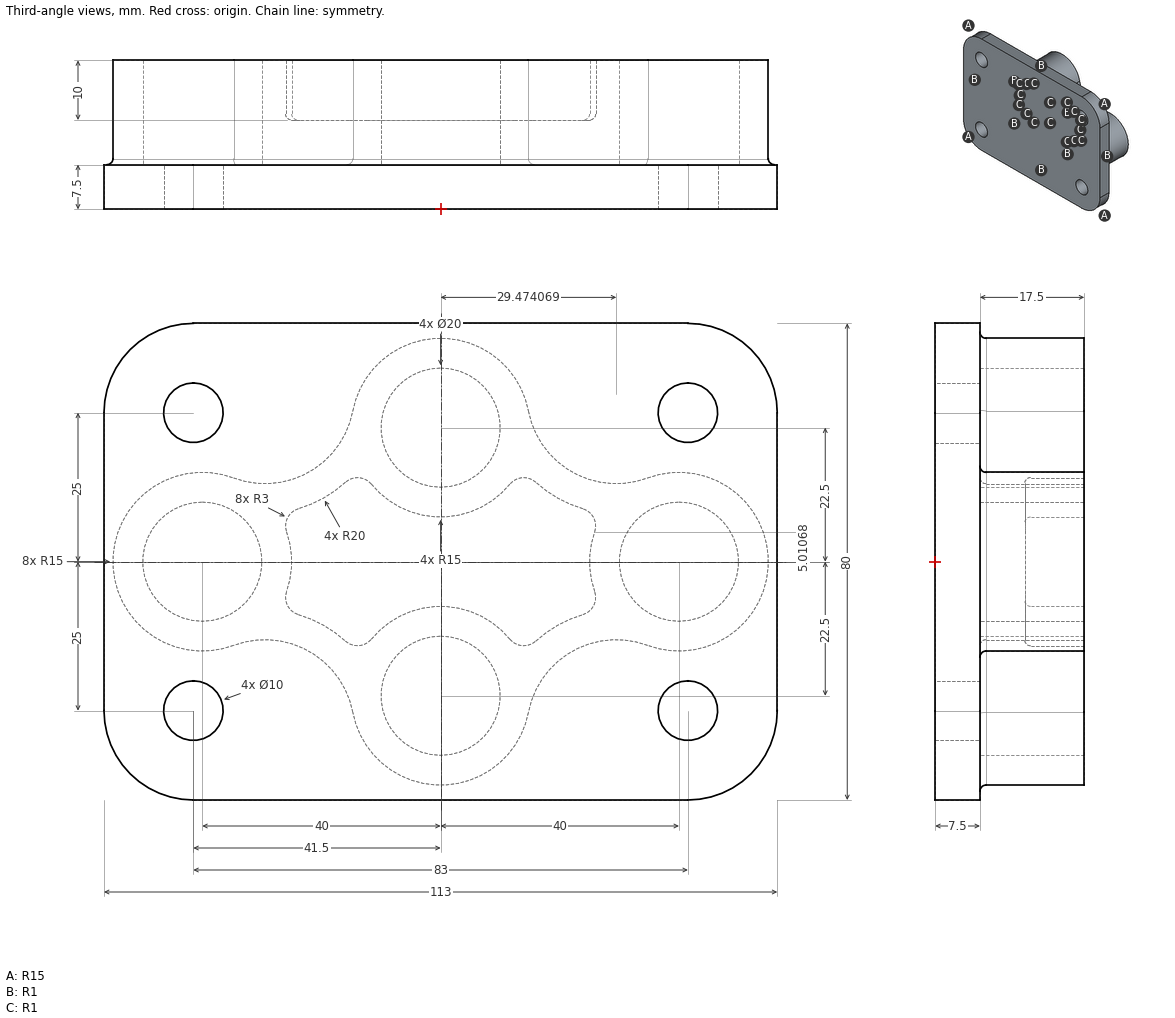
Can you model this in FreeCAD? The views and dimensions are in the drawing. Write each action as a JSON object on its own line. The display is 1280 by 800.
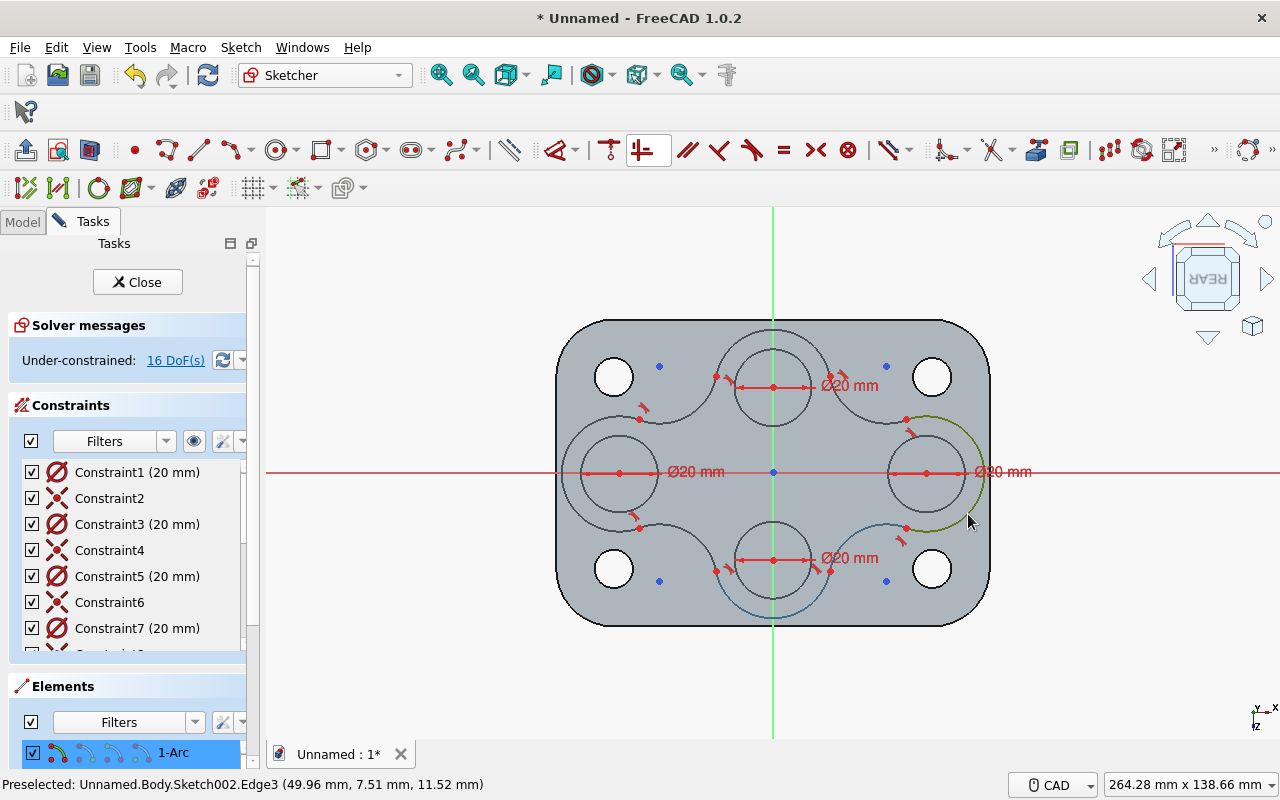
{"action": "left_click", "coordinate": [843, 404]}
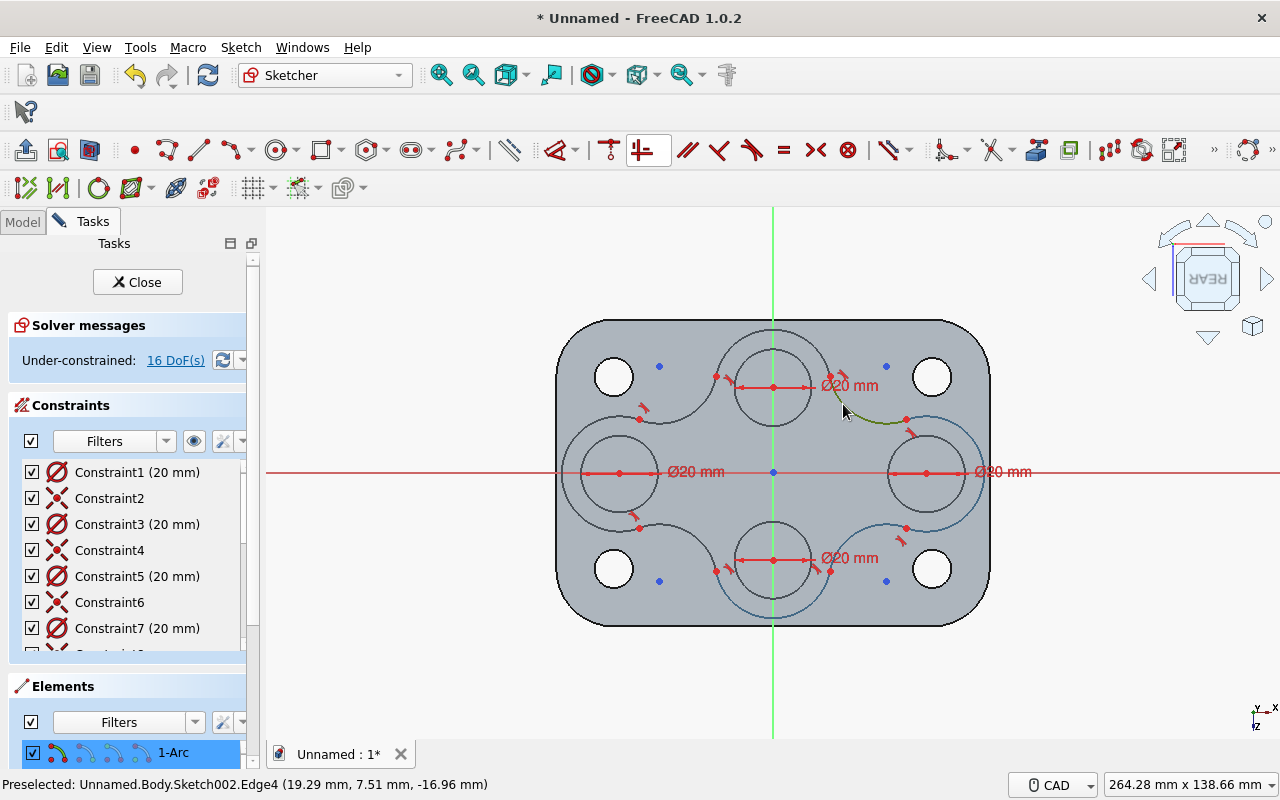
{"action": "left_click", "coordinate": [803, 338]}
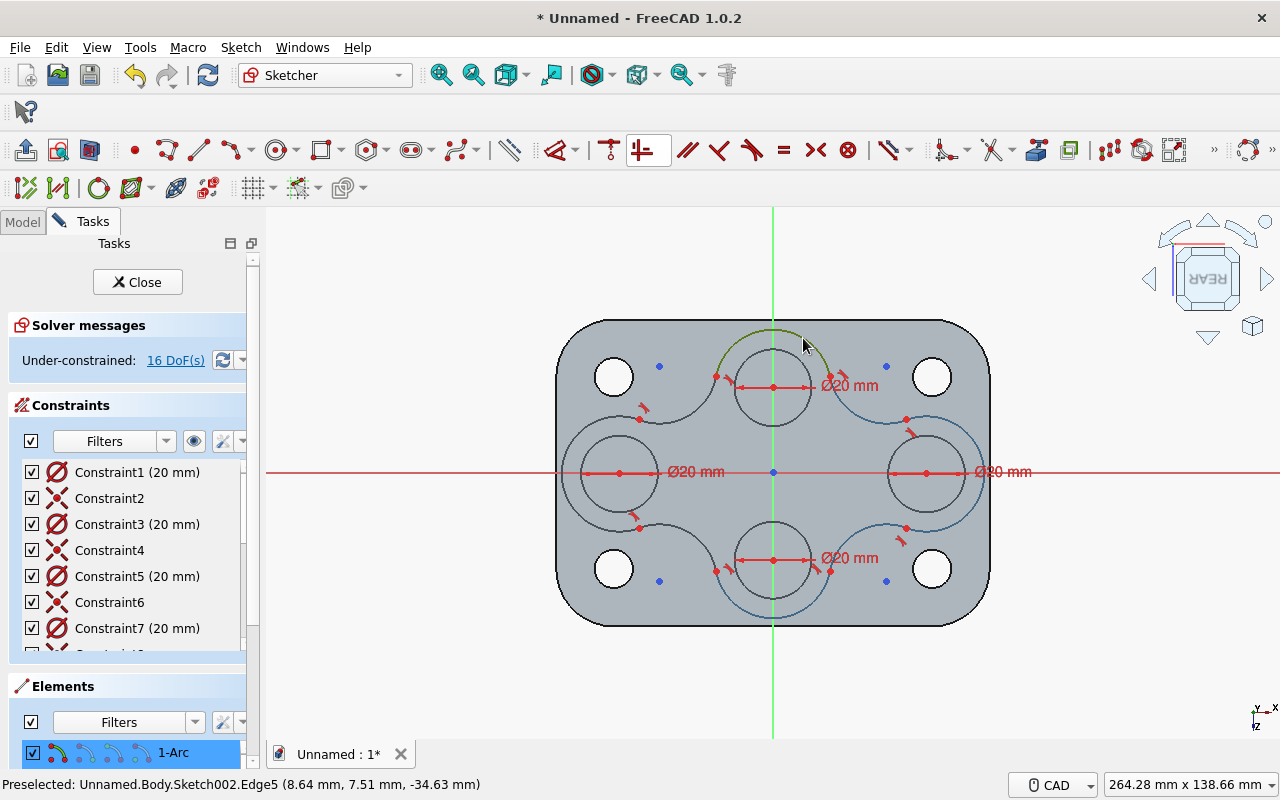
{"action": "left_click", "coordinate": [669, 423]}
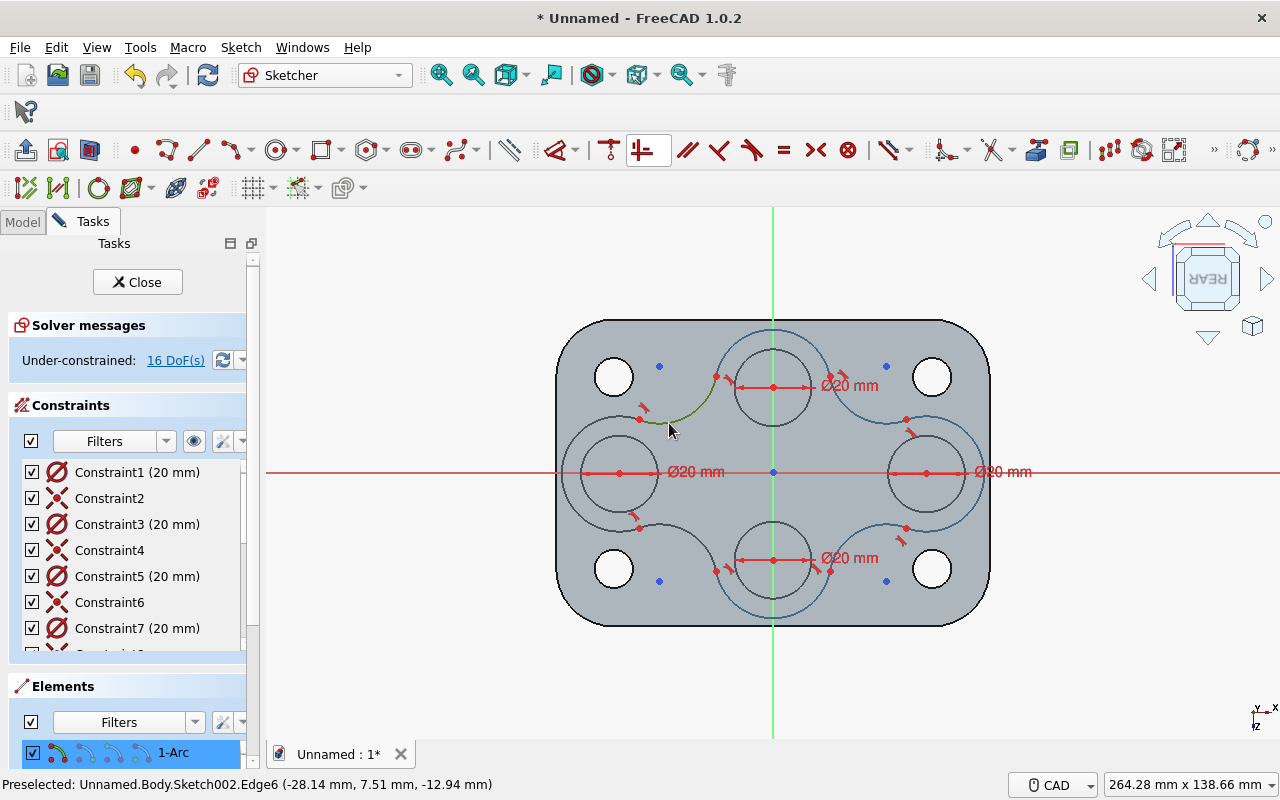
{"action": "left_click", "coordinate": [578, 434]}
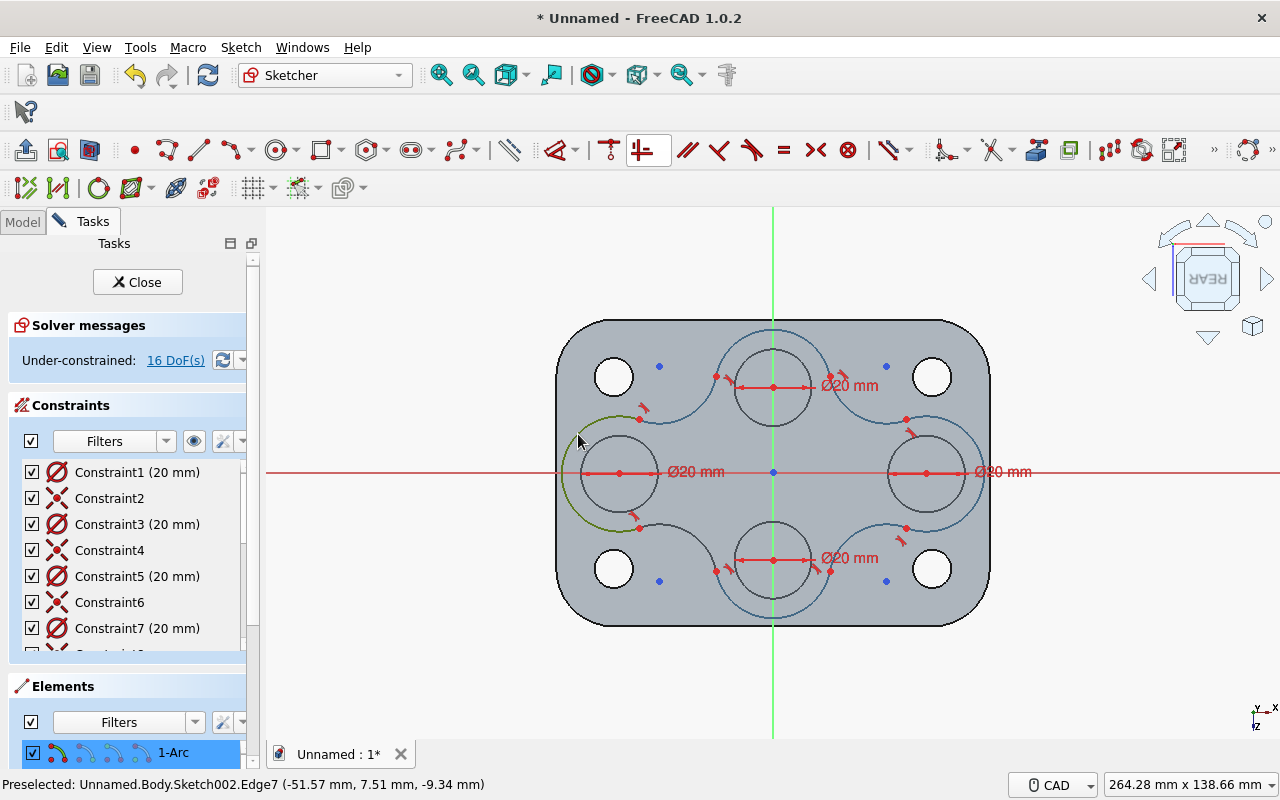
{"action": "left_click", "coordinate": [703, 544]}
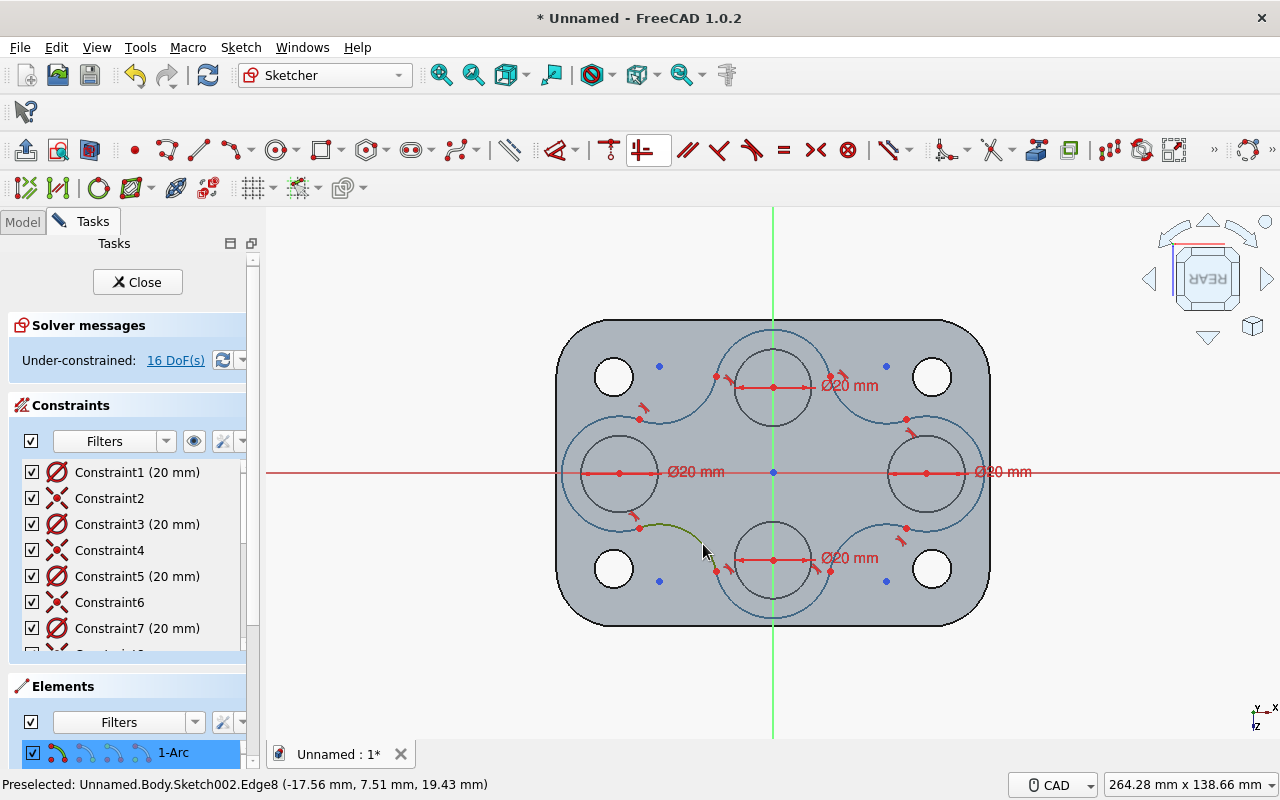
{"action": "left_click", "coordinate": [784, 150]}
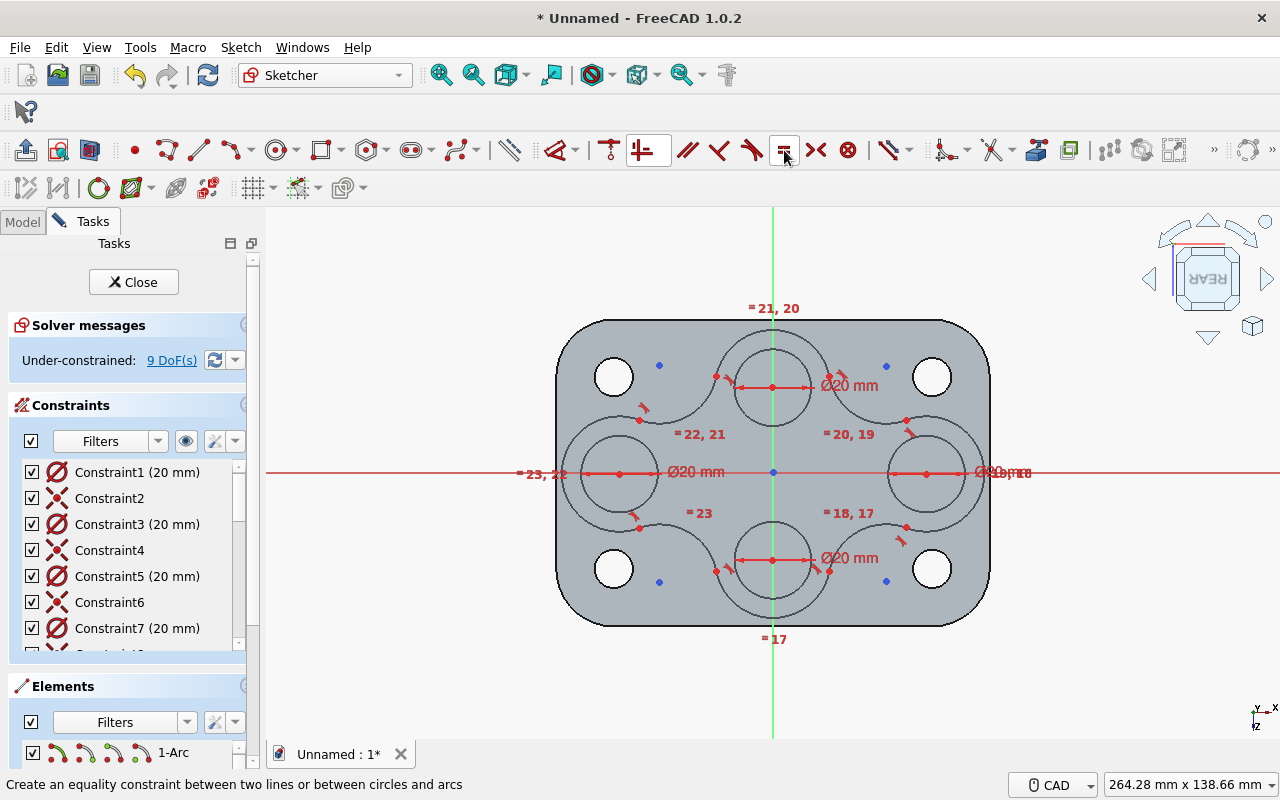
{"action": "left_click", "coordinate": [773, 560]}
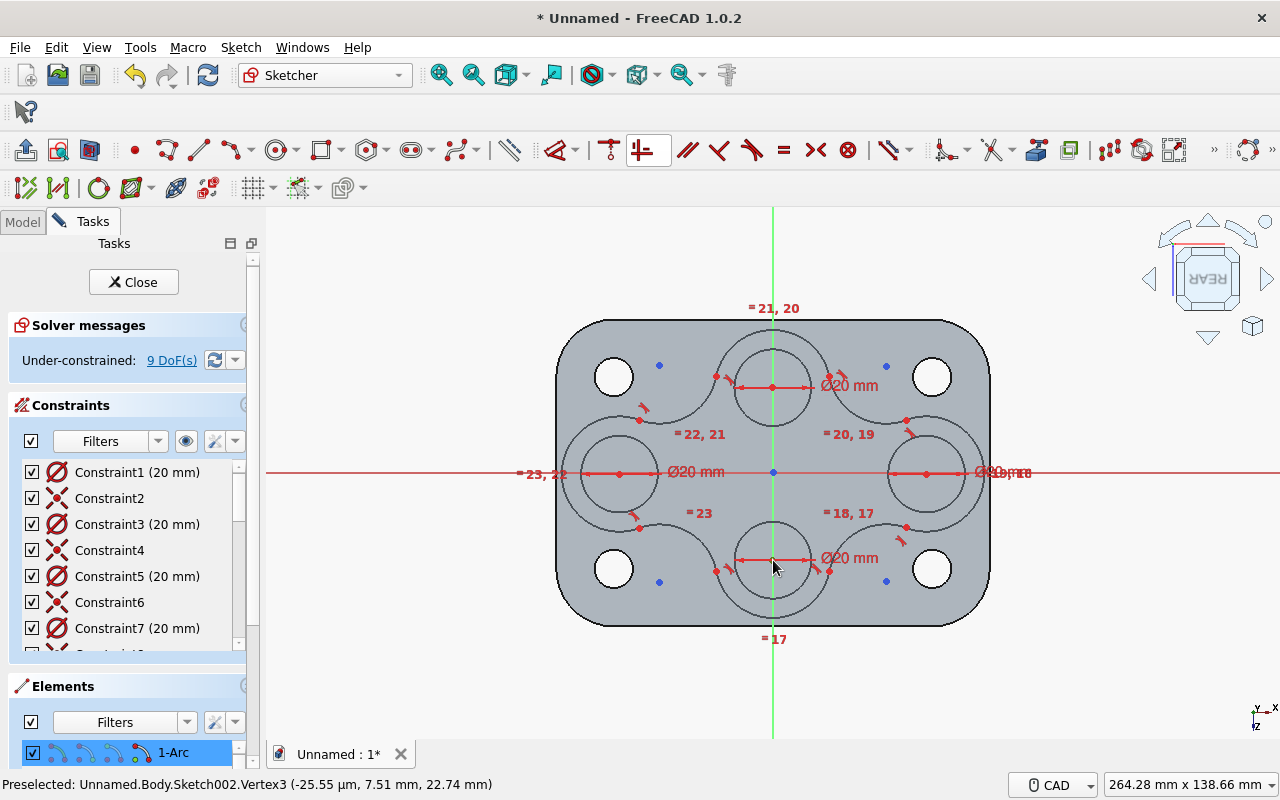
{"action": "left_click", "coordinate": [773, 677]}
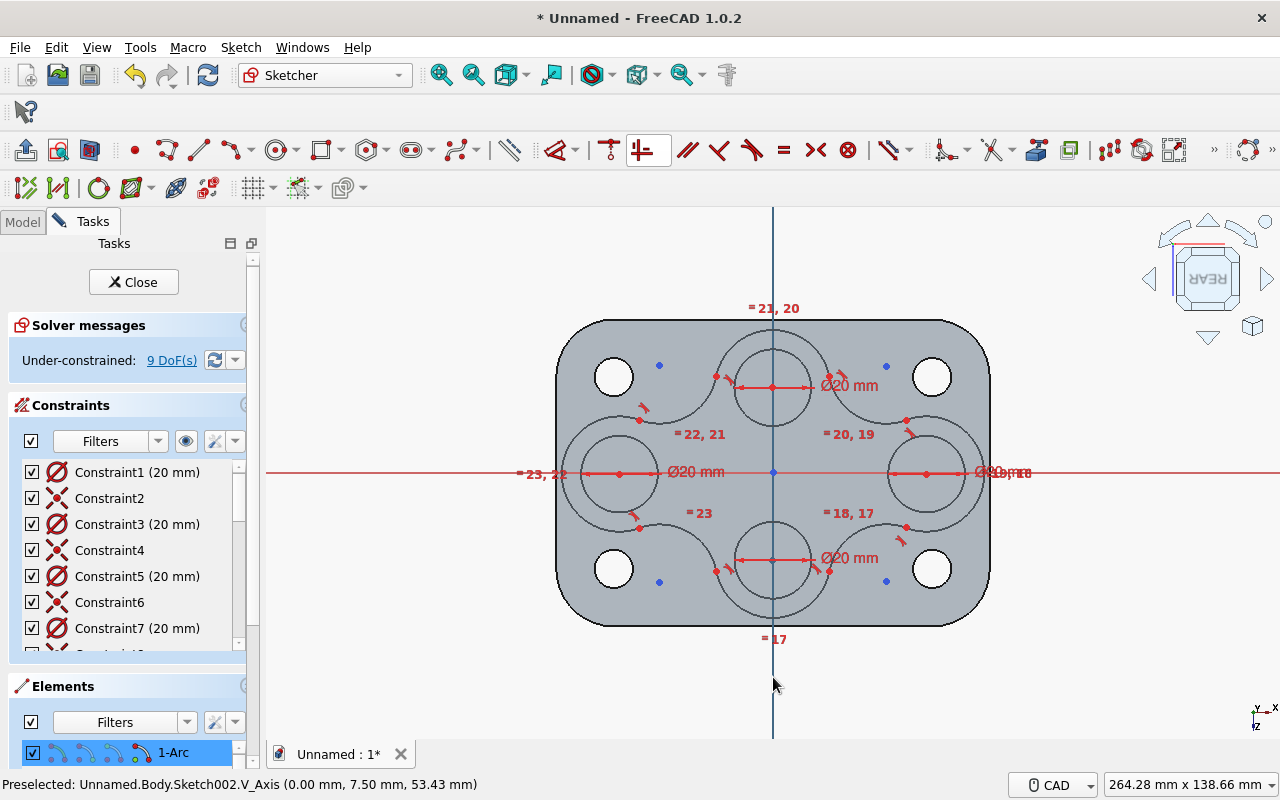
{"action": "key", "text": "c"}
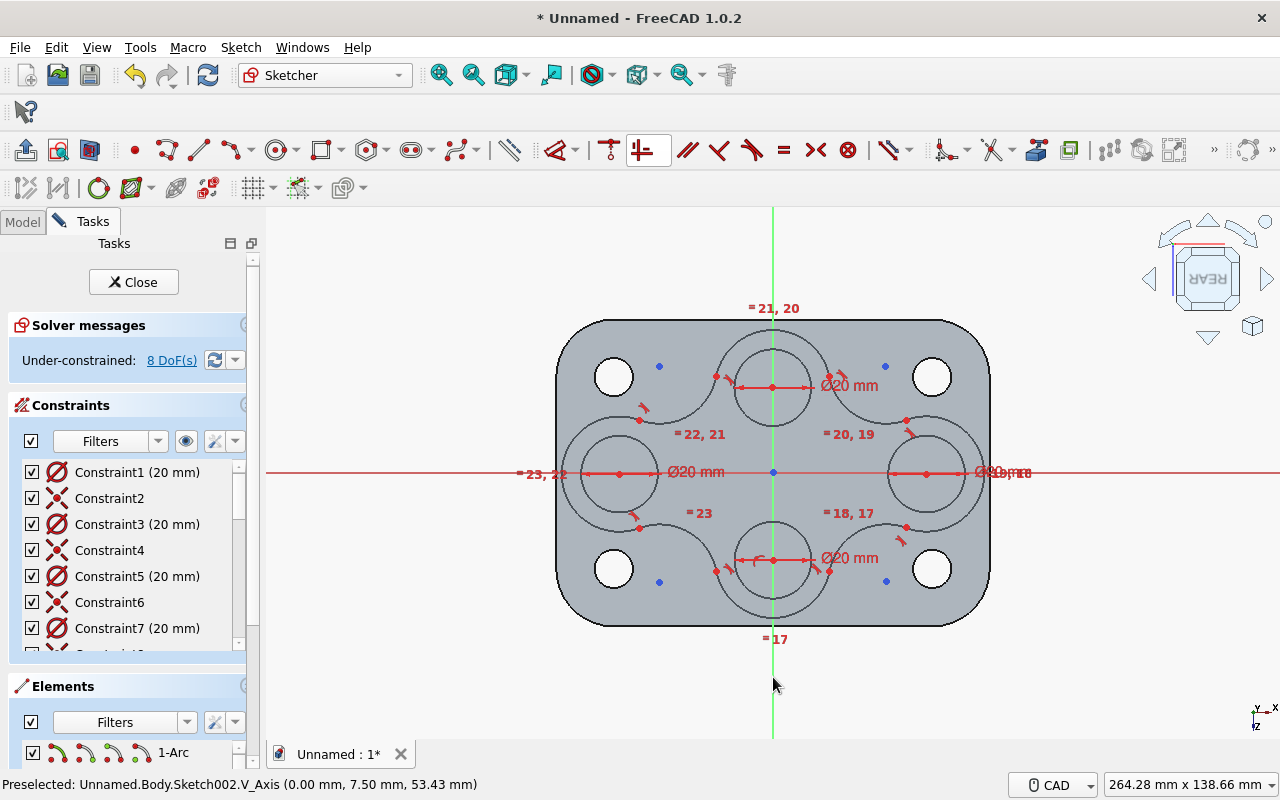
{"action": "left_click", "coordinate": [927, 474]}